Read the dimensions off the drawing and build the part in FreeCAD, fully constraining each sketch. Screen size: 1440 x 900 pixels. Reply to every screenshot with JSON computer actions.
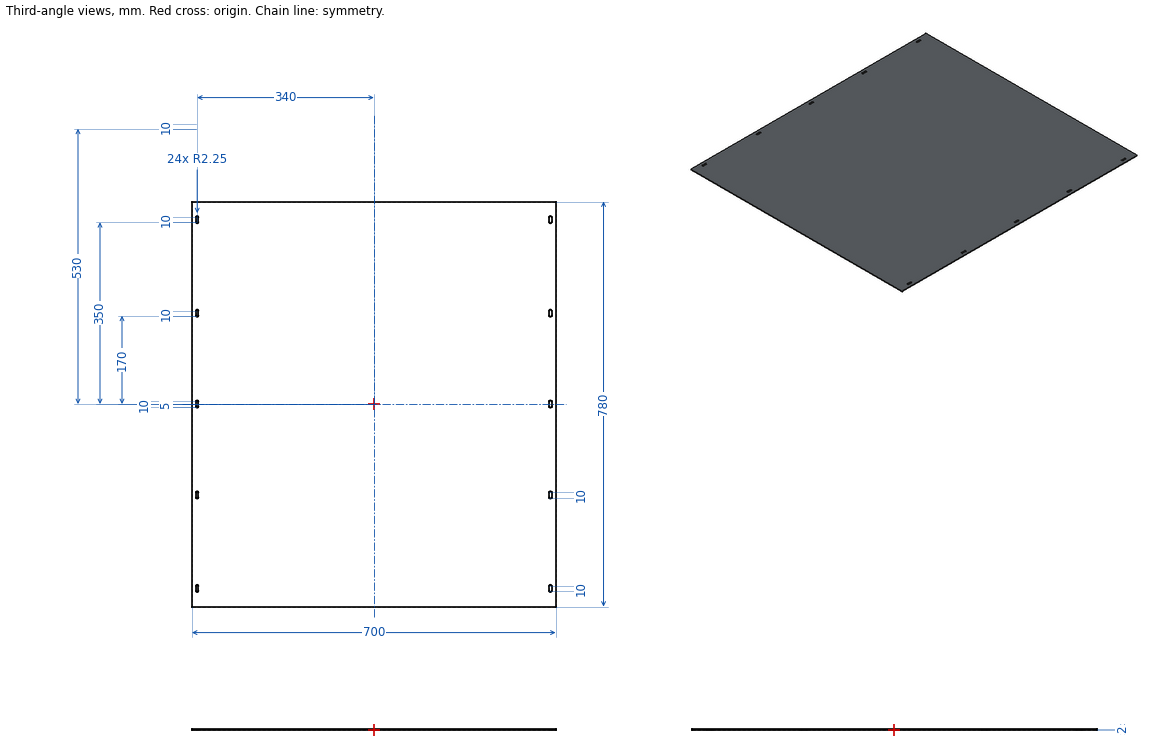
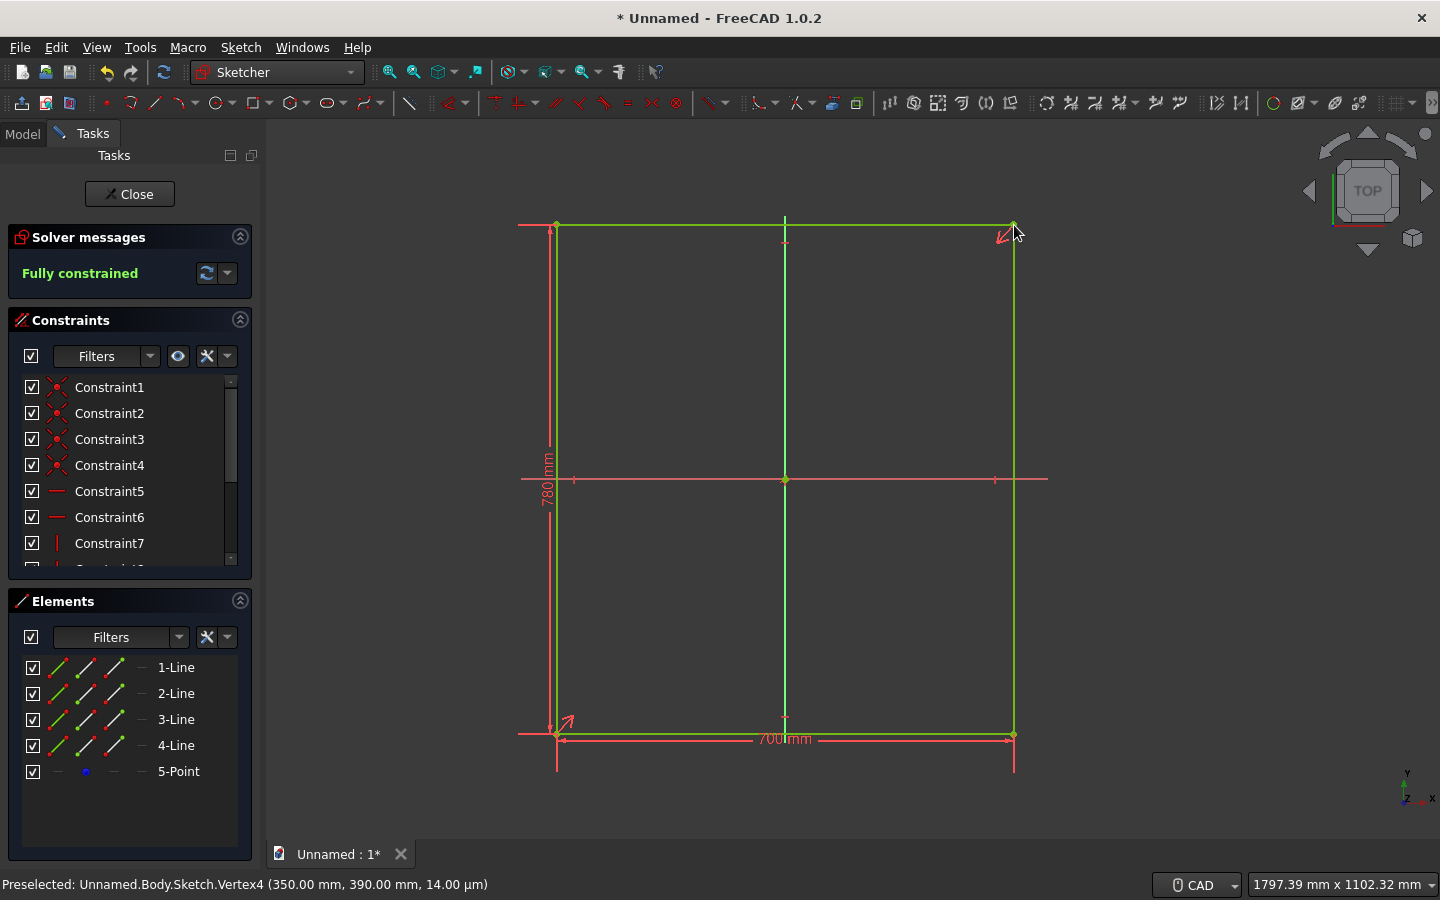
{"action": "left_click", "coordinate": [130, 194]}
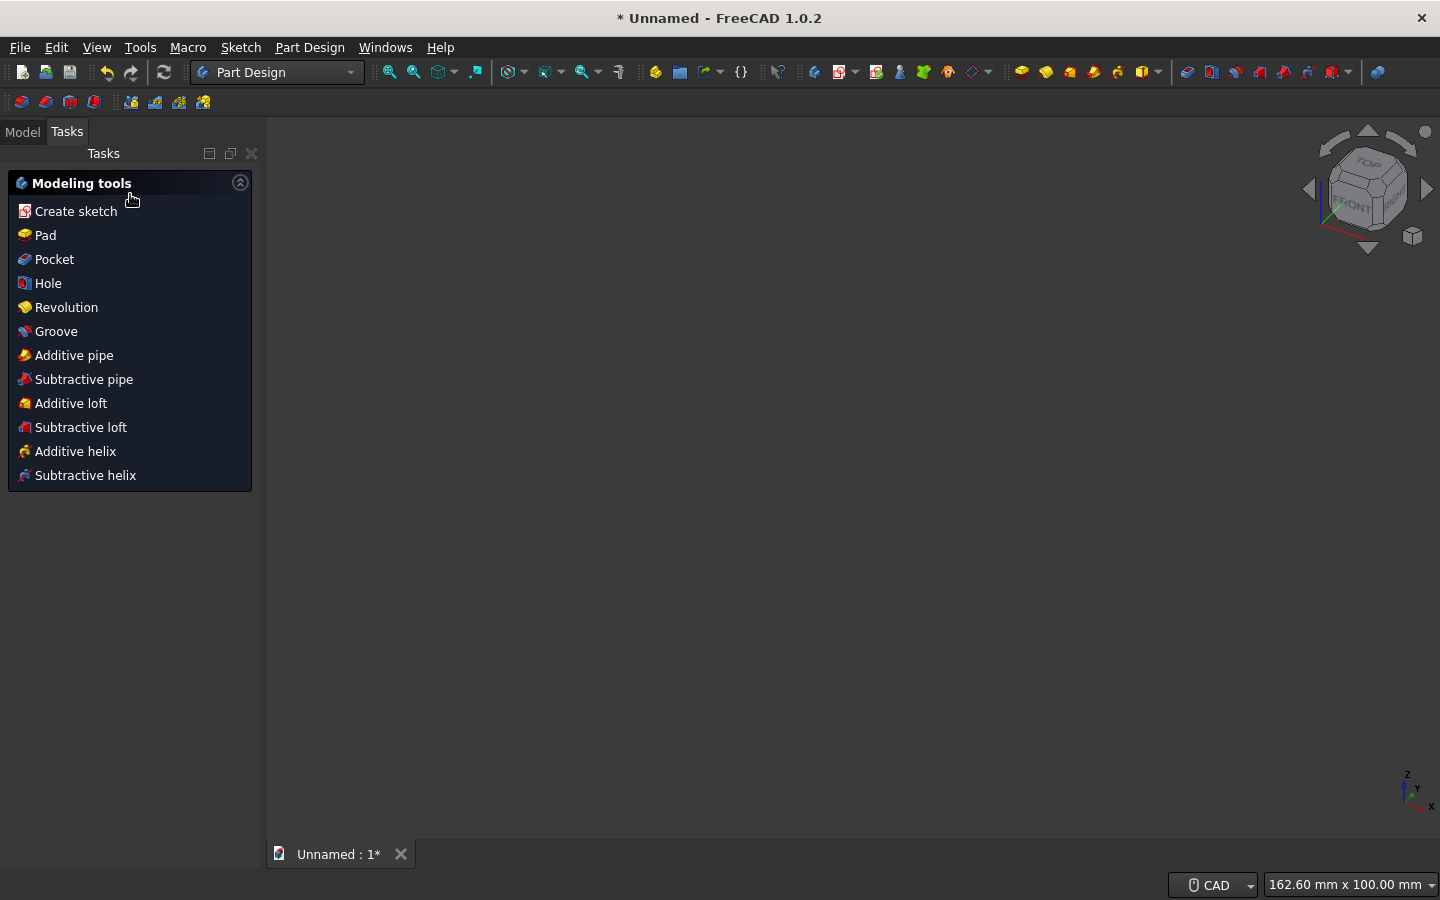
{"action": "left_click", "coordinate": [1022, 72]}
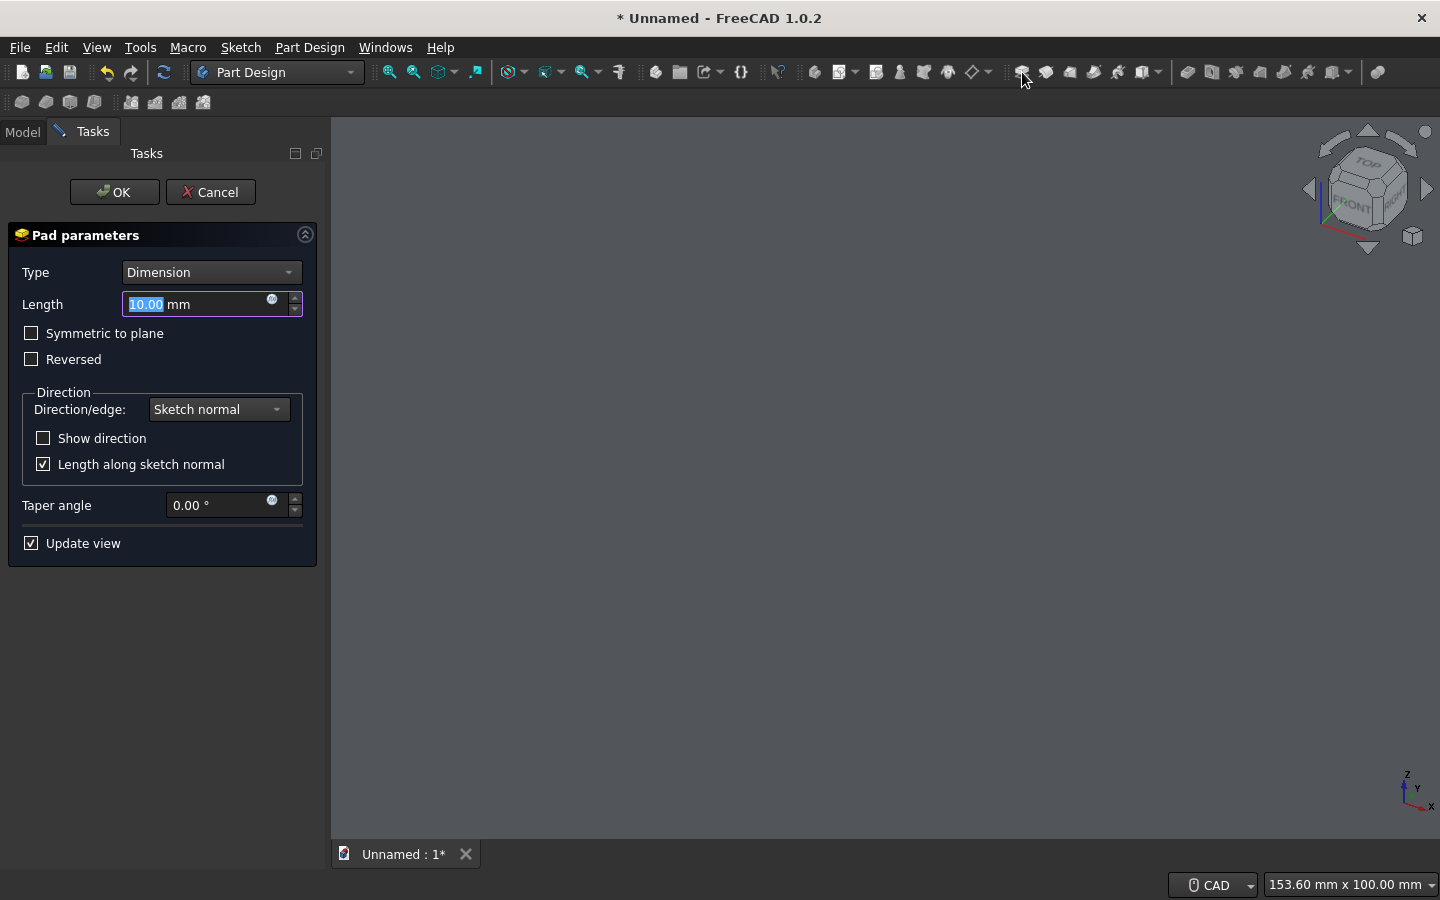
{"action": "type", "text": "2"}
{"action": "key", "text": "Tab"}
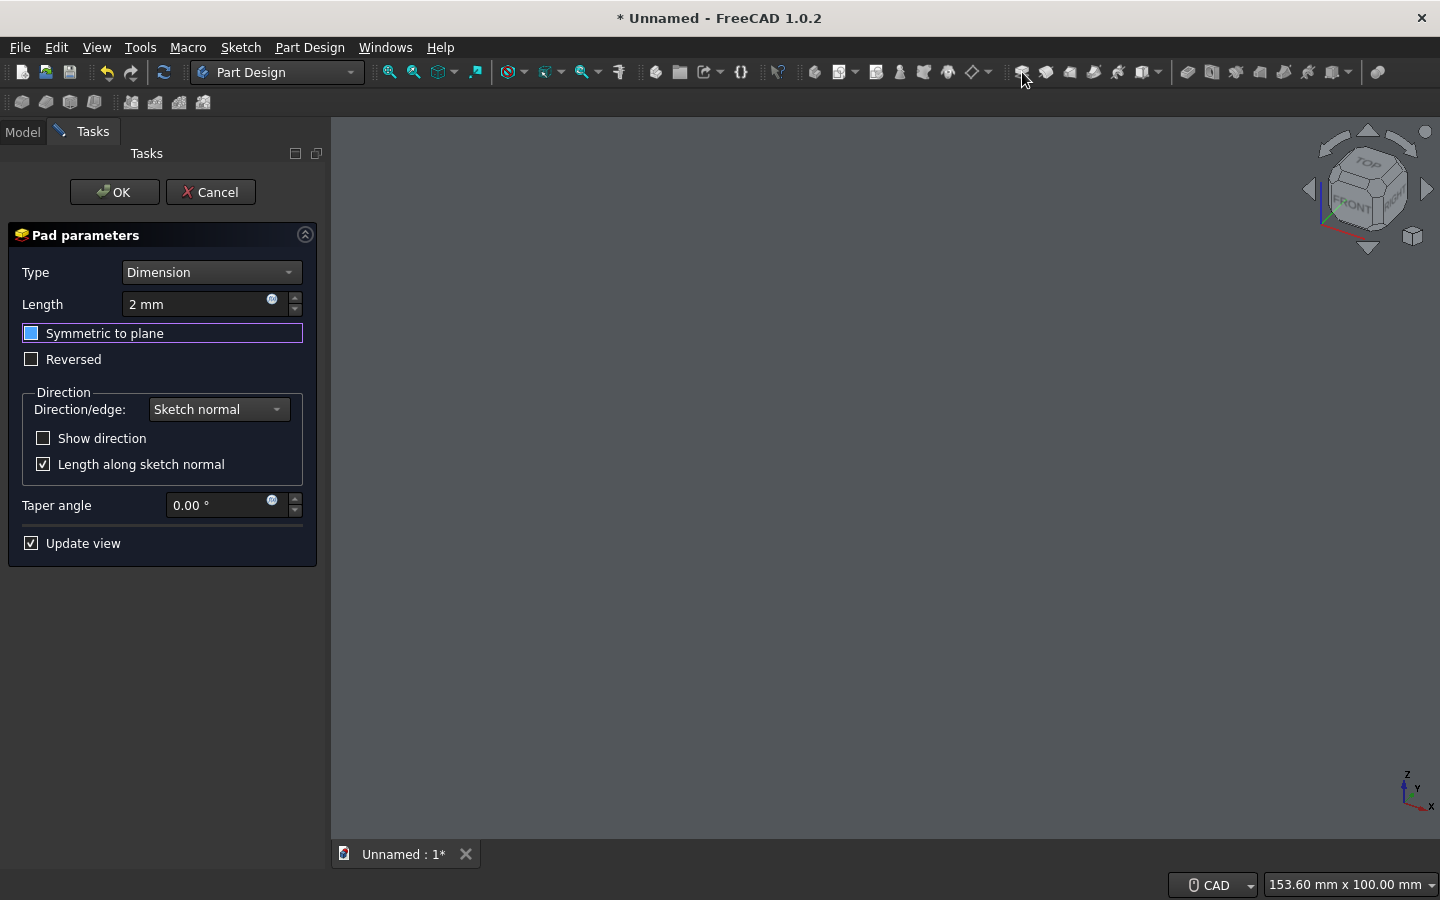
{"action": "left_click", "coordinate": [115, 192]}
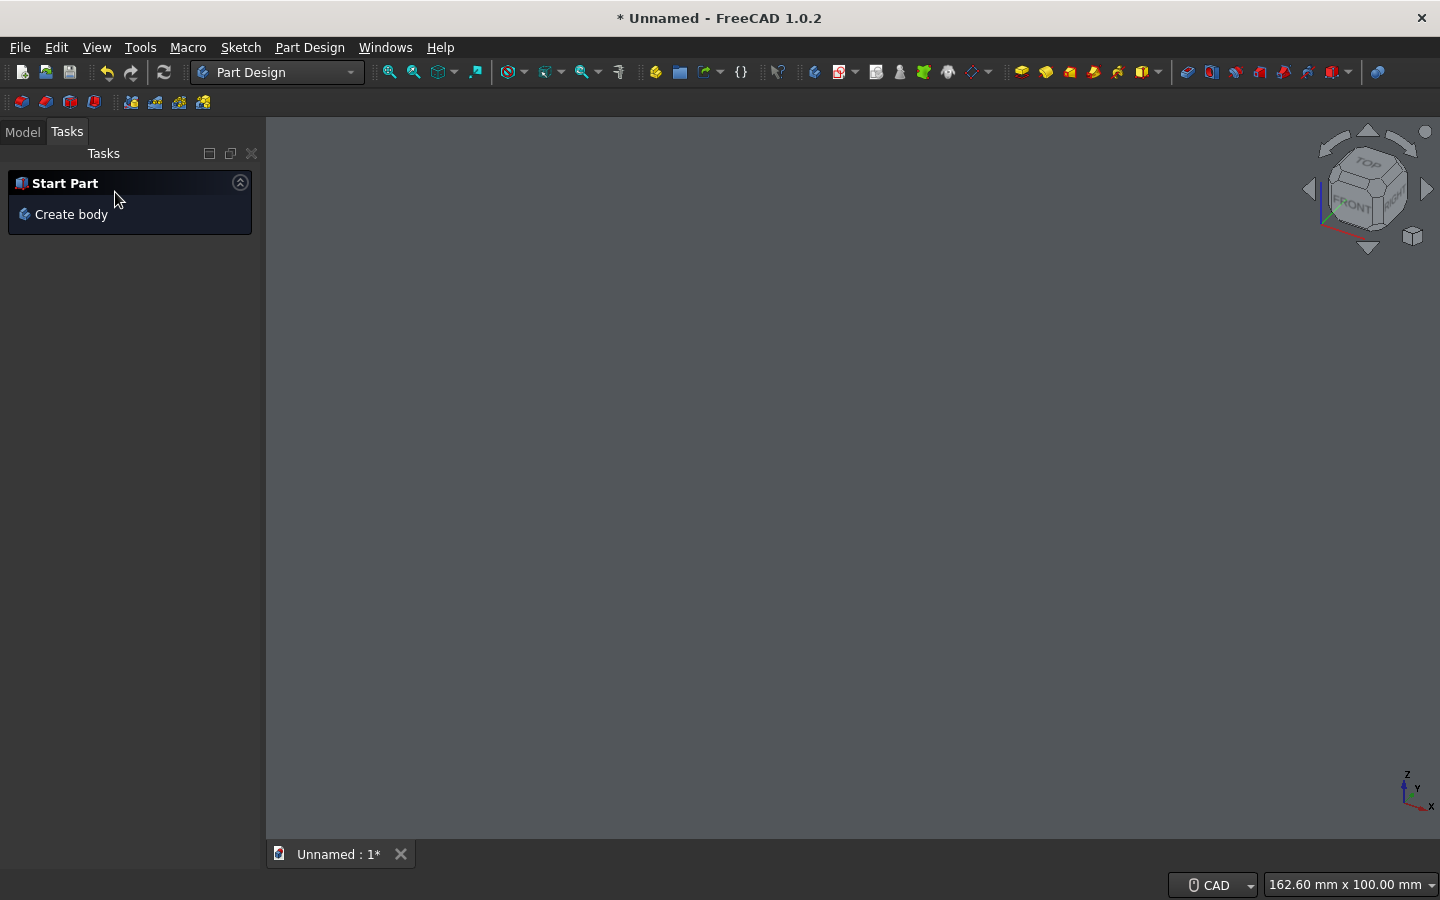
{"action": "key", "text": "v f"}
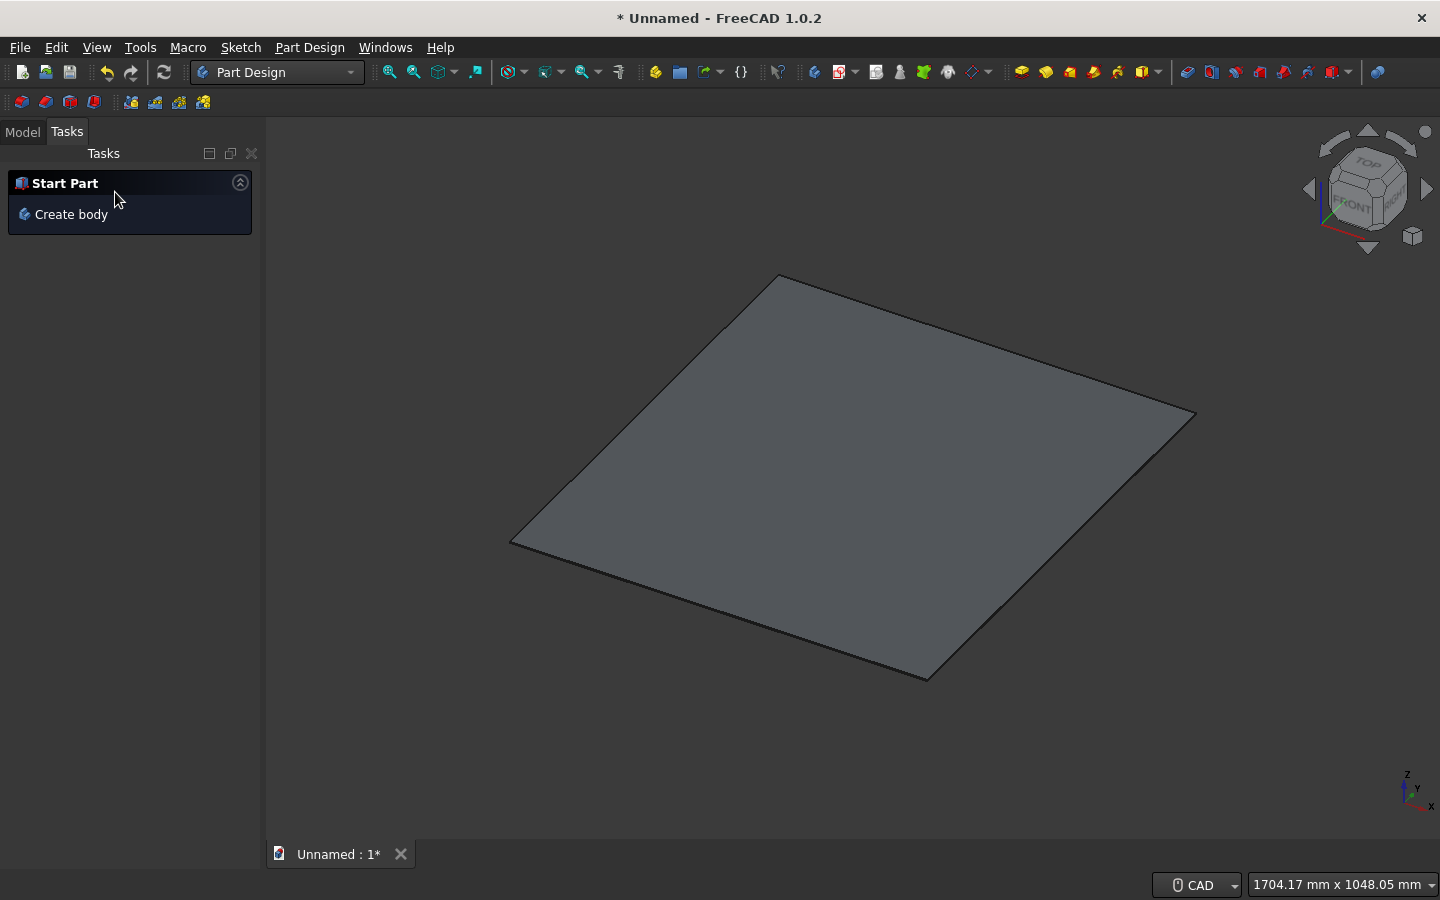
{"action": "left_click", "coordinate": [853, 476]}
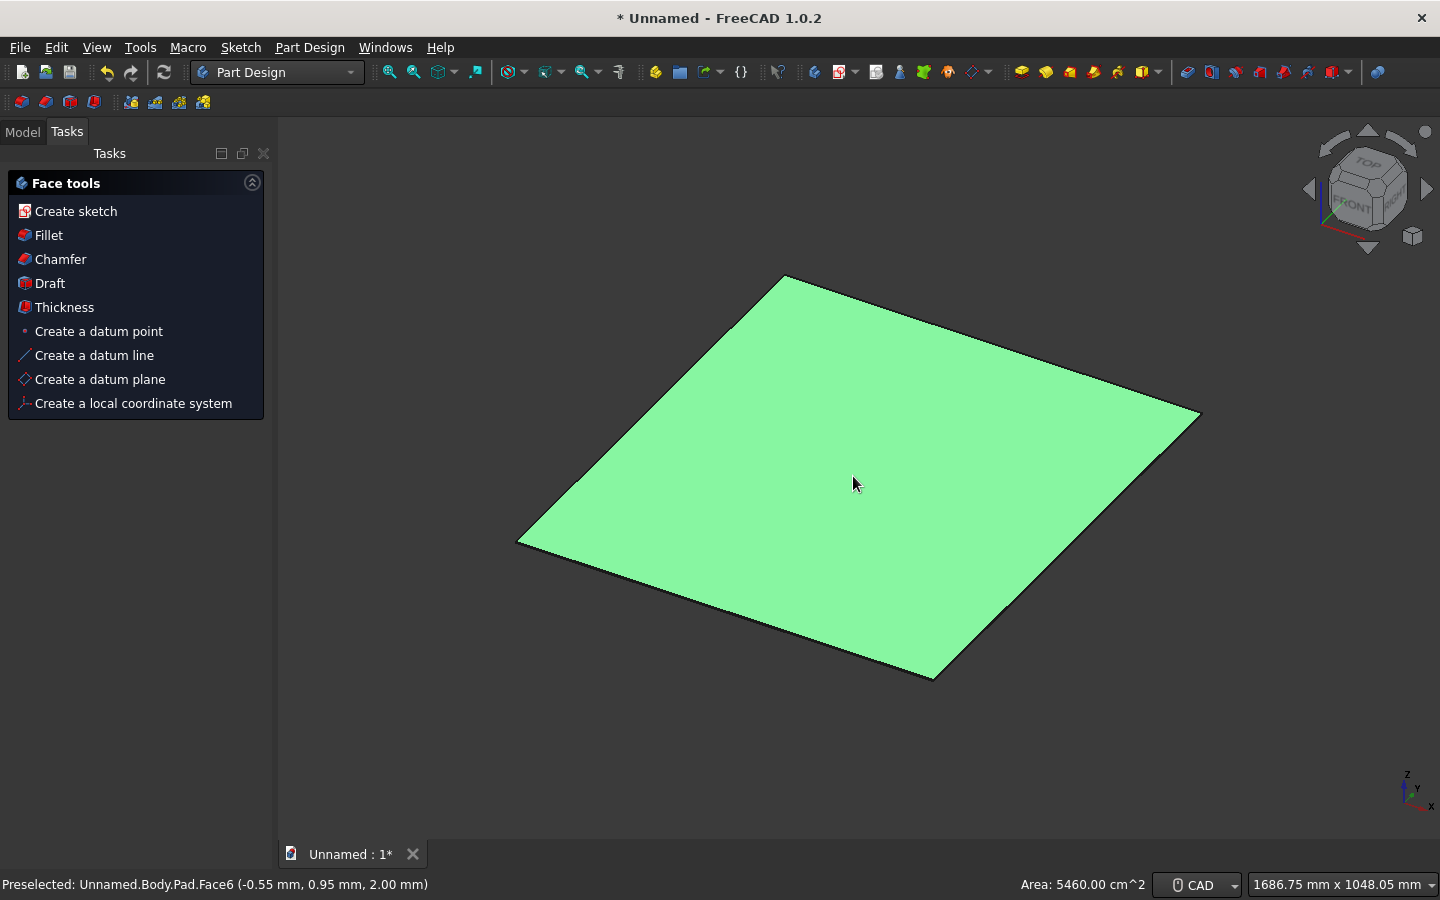
{"action": "left_click", "coordinate": [840, 72]}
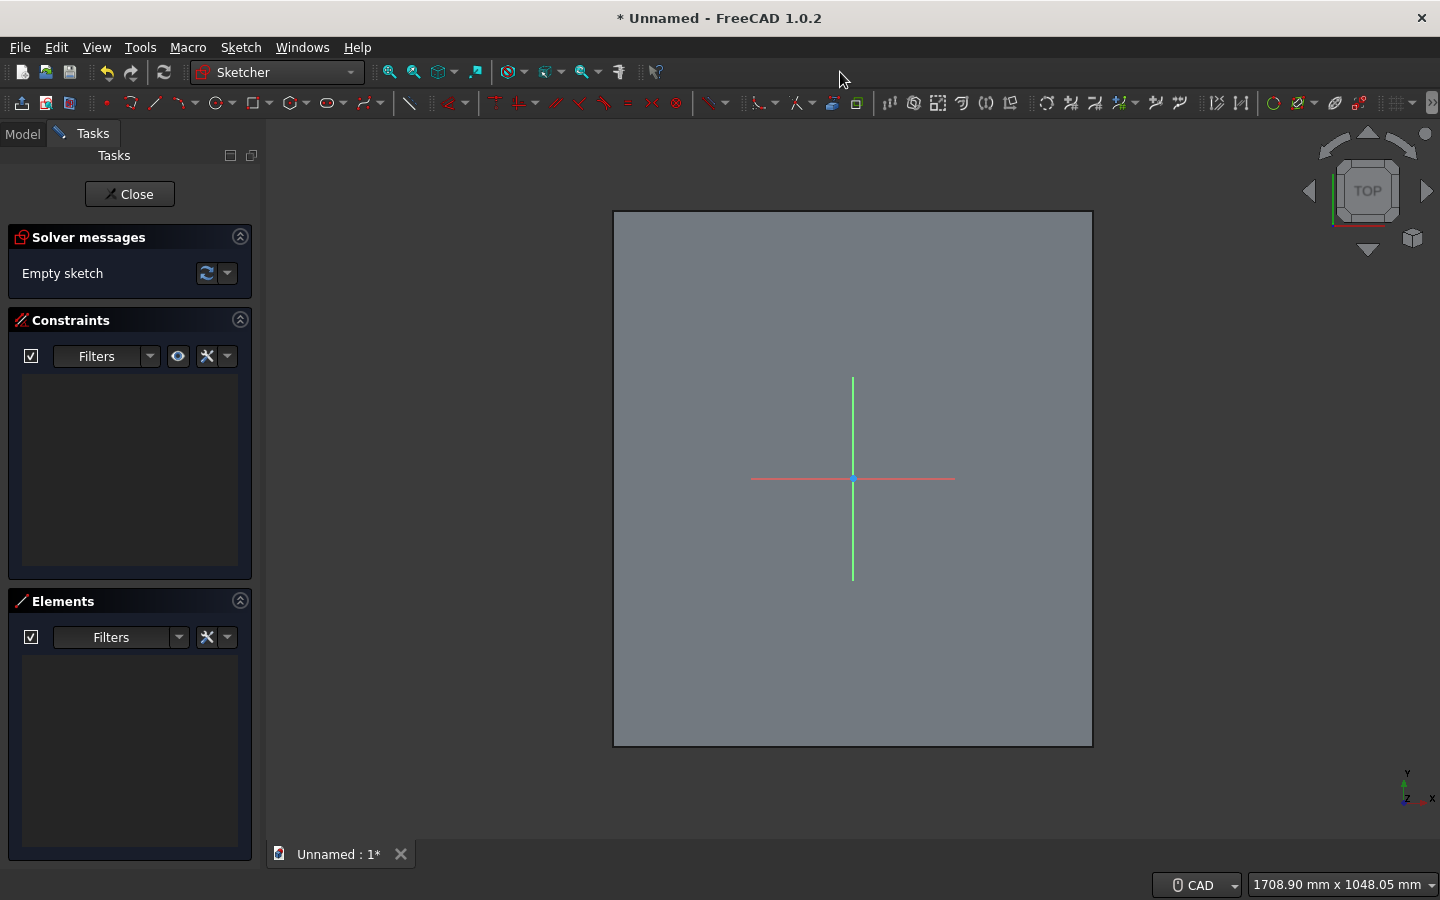
{"action": "scroll", "coordinate": [475, 758], "scroll_direction": "down", "scroll_amount": 1}